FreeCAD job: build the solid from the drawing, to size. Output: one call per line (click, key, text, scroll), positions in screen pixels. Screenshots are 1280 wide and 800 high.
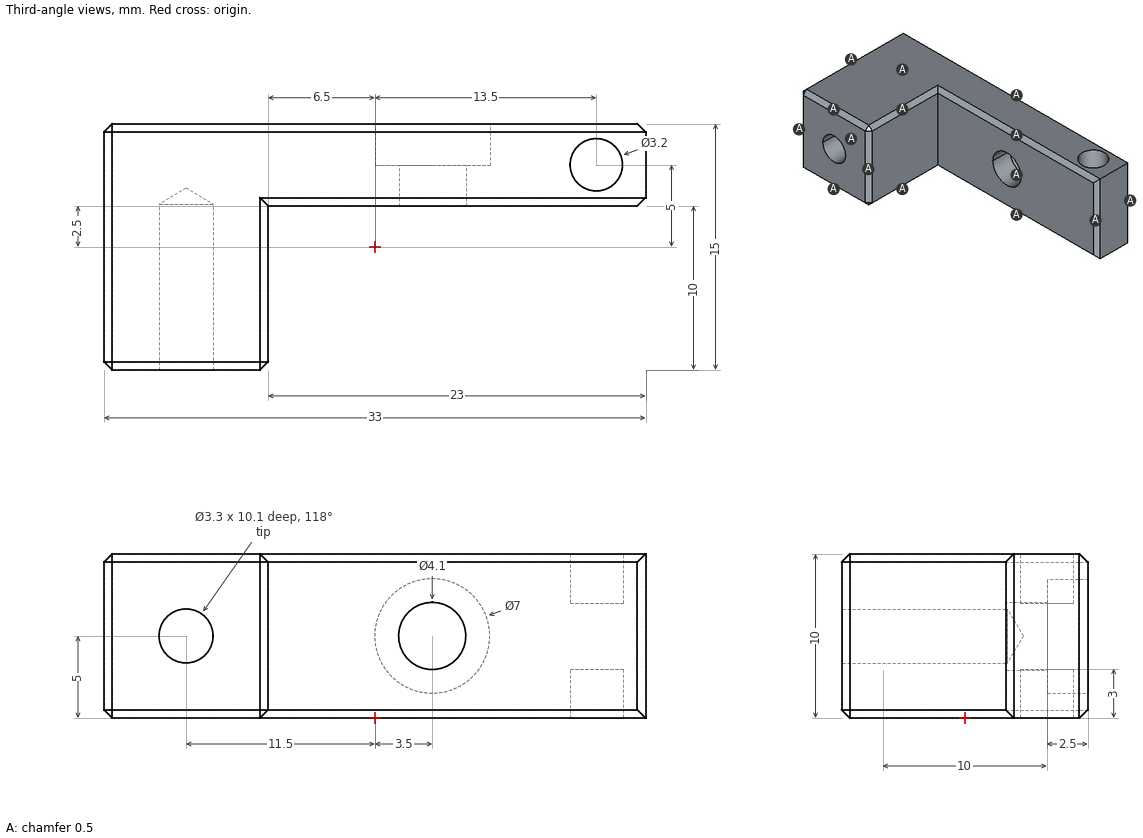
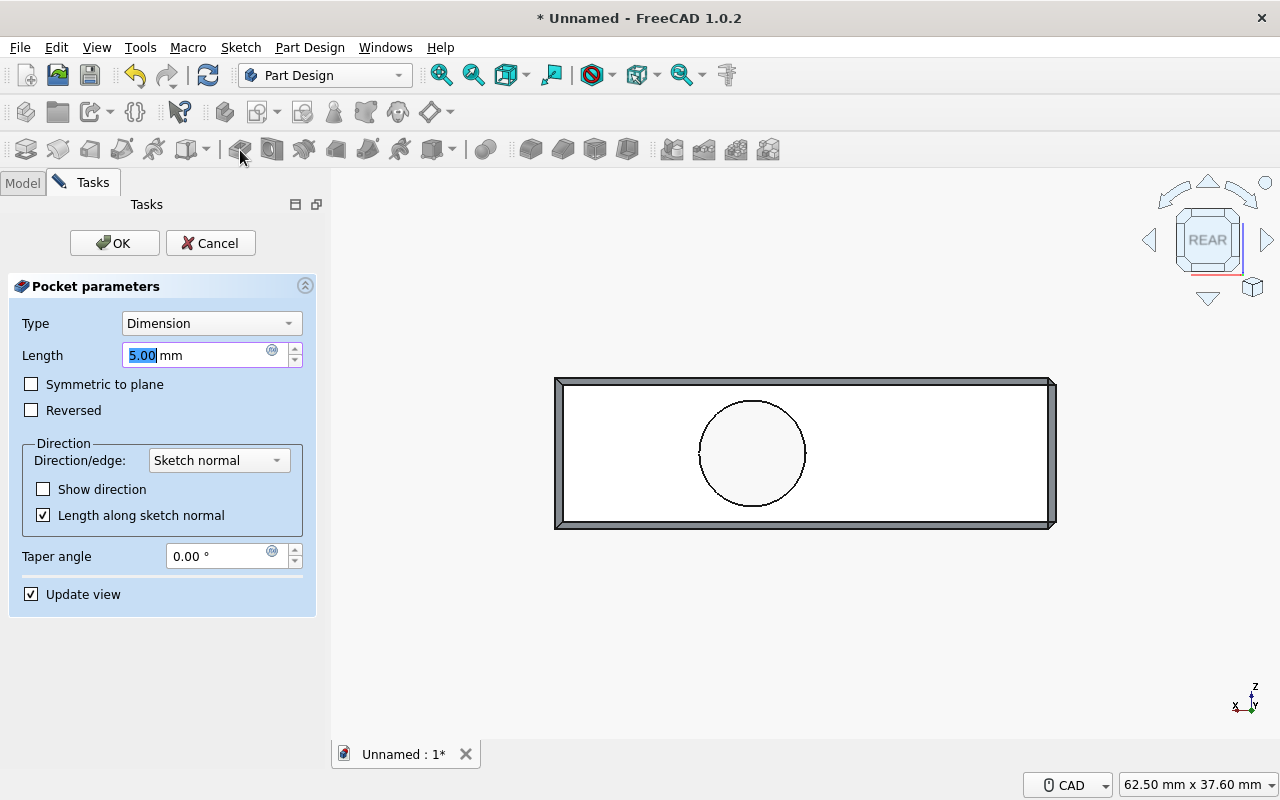
text(2.5)
key(Tab)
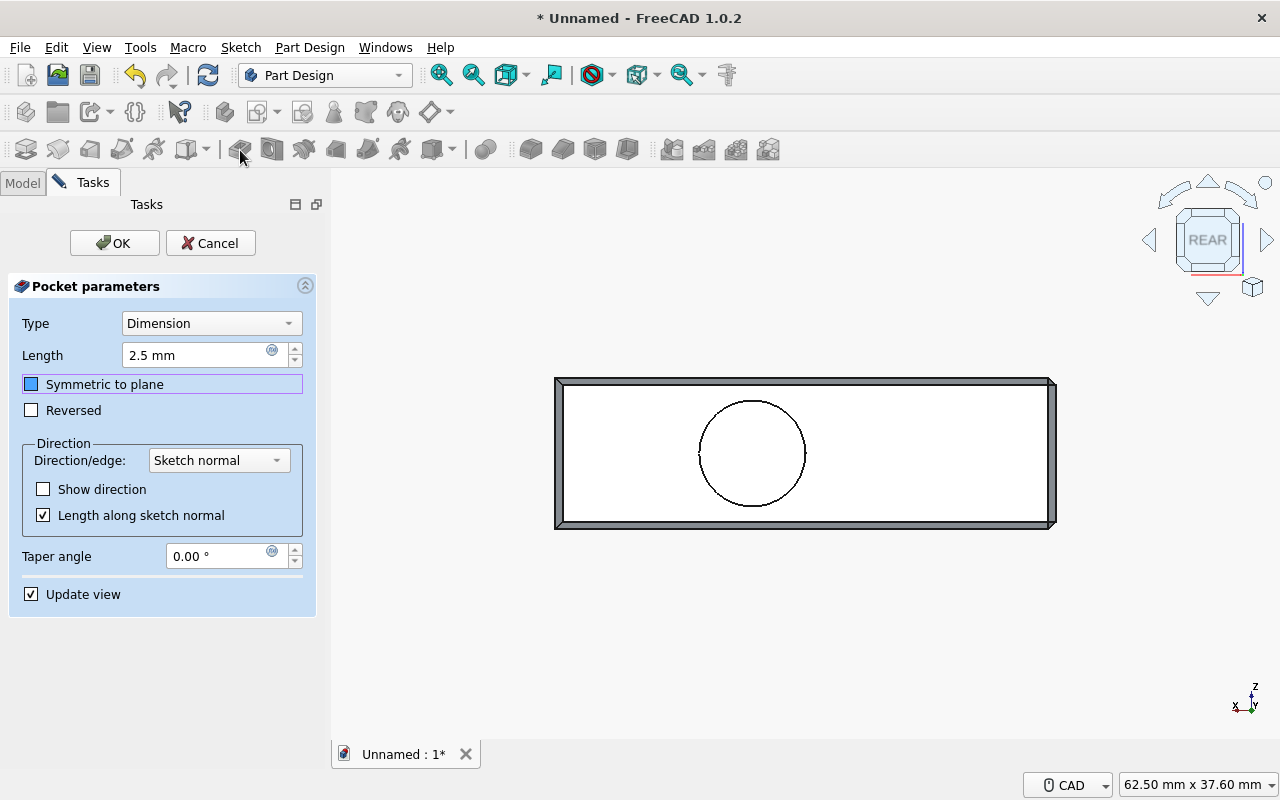
click(115, 243)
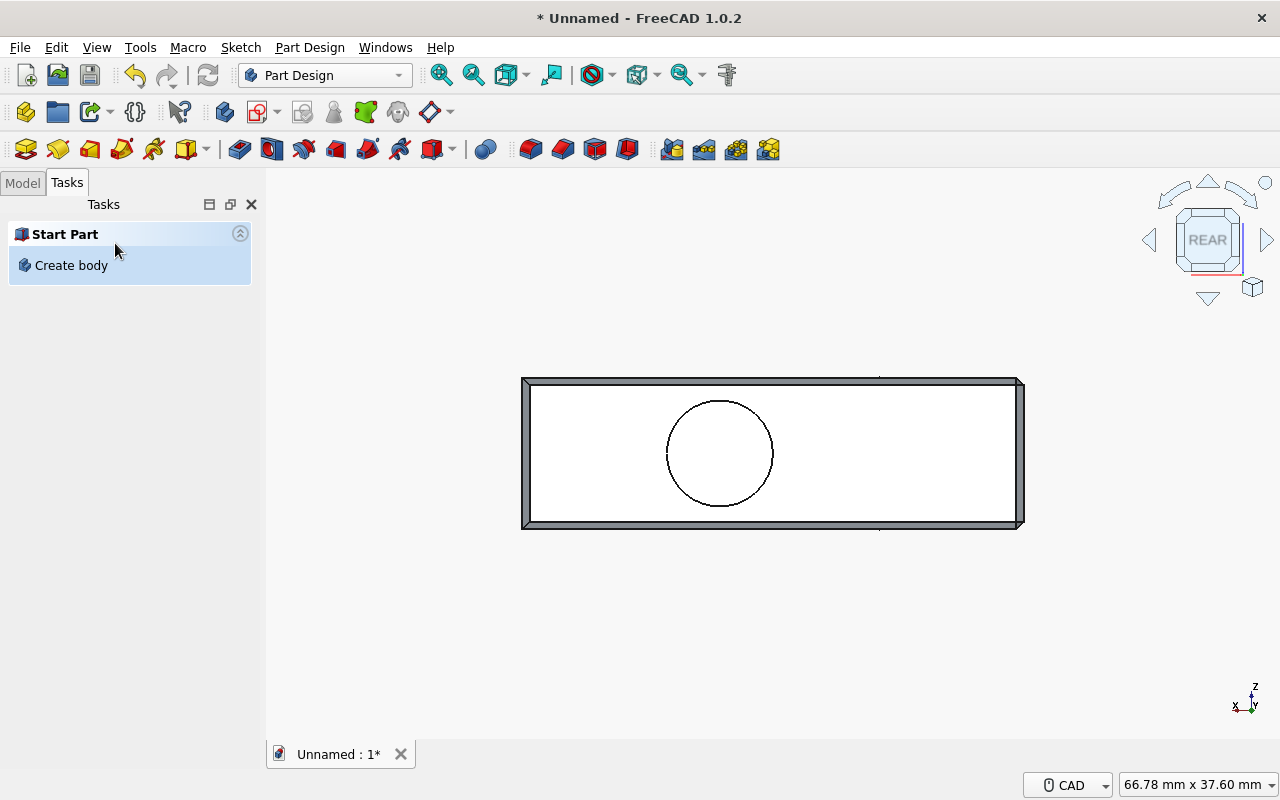
click(258, 112)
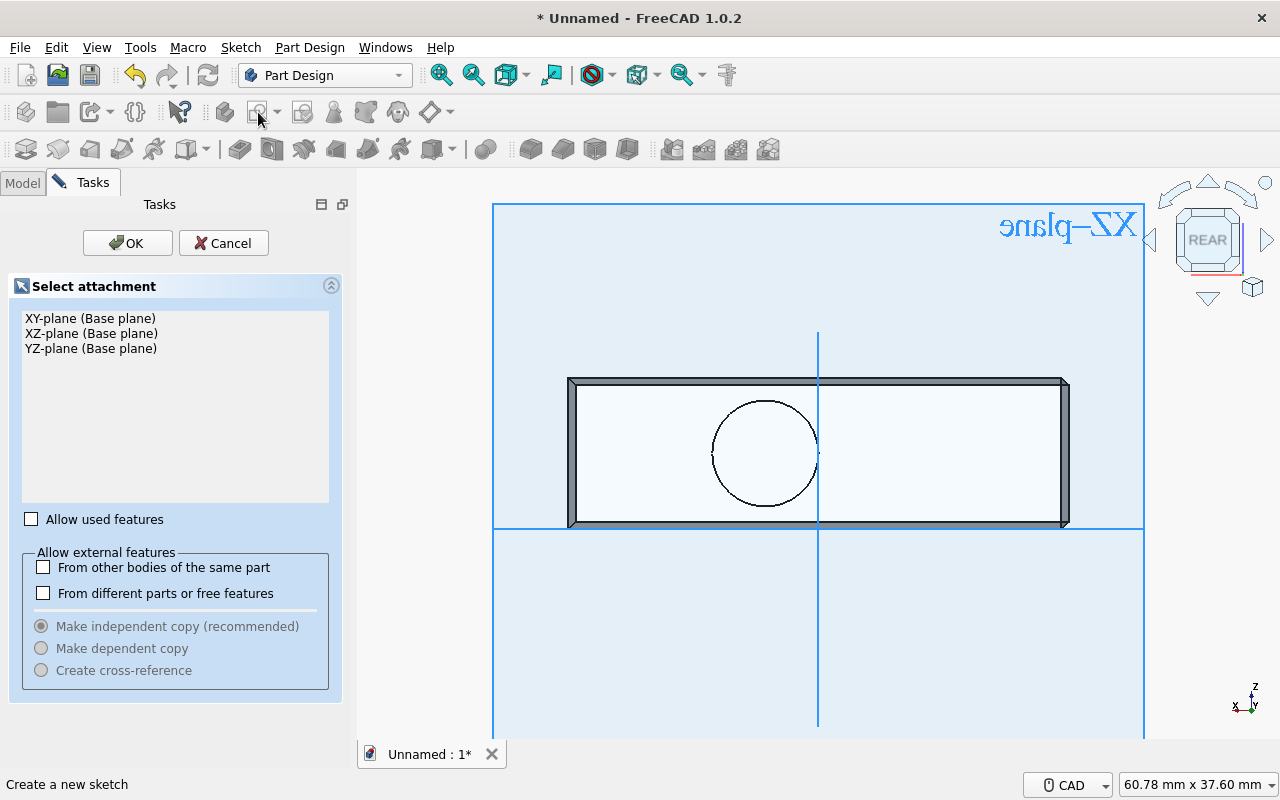
click(82, 318)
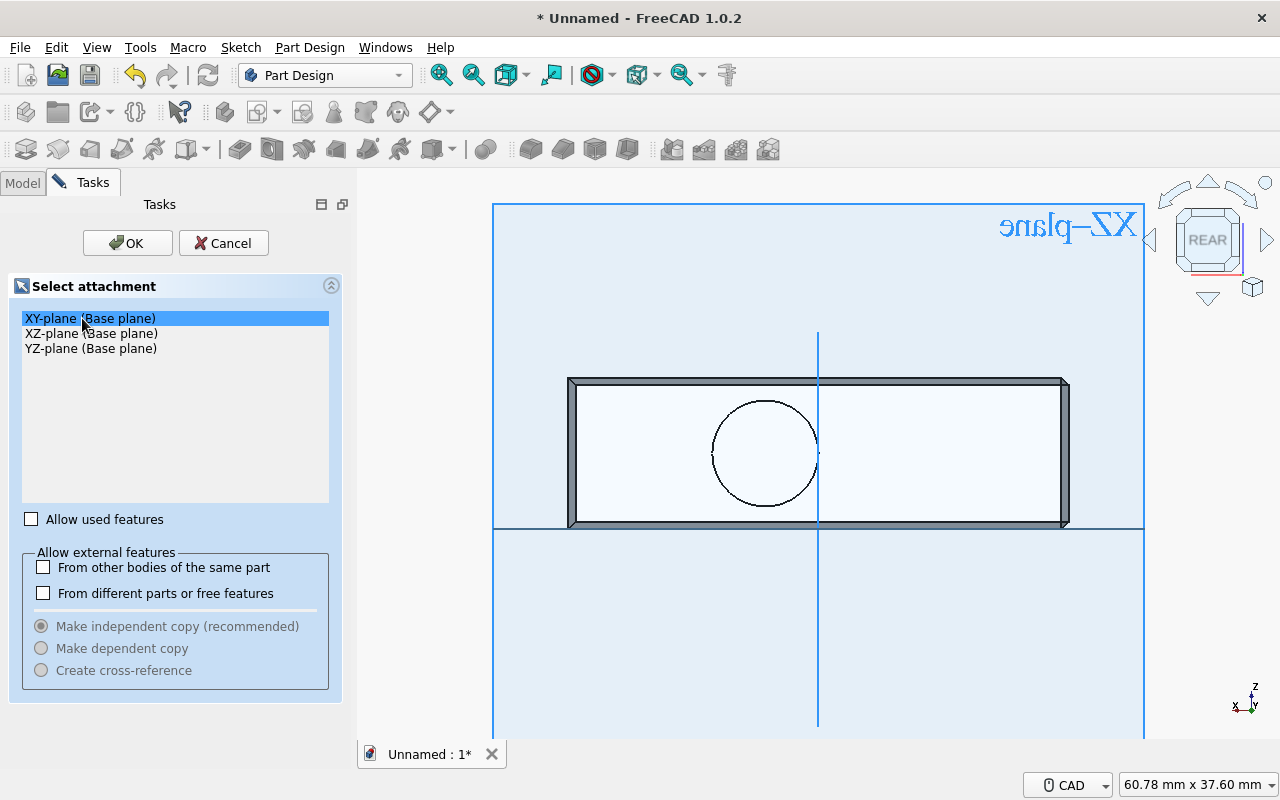
click(128, 243)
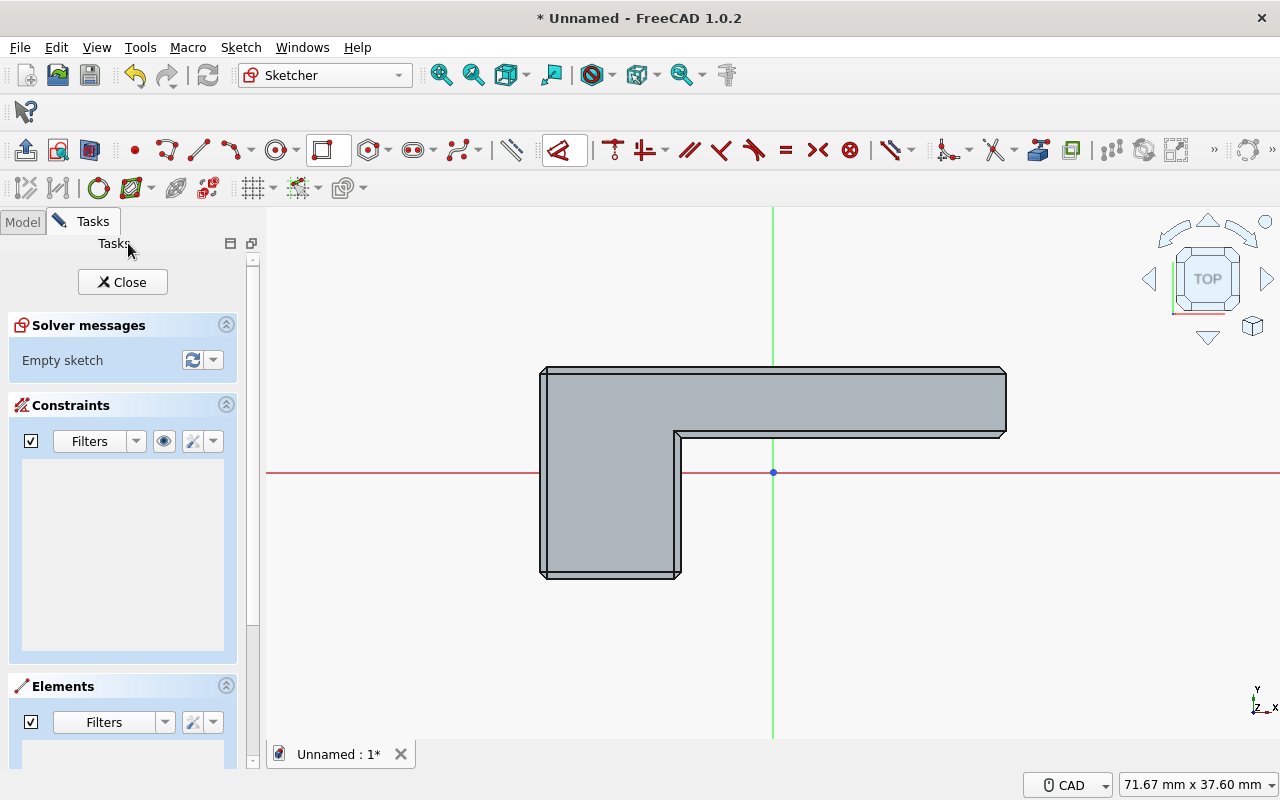
click(90, 150)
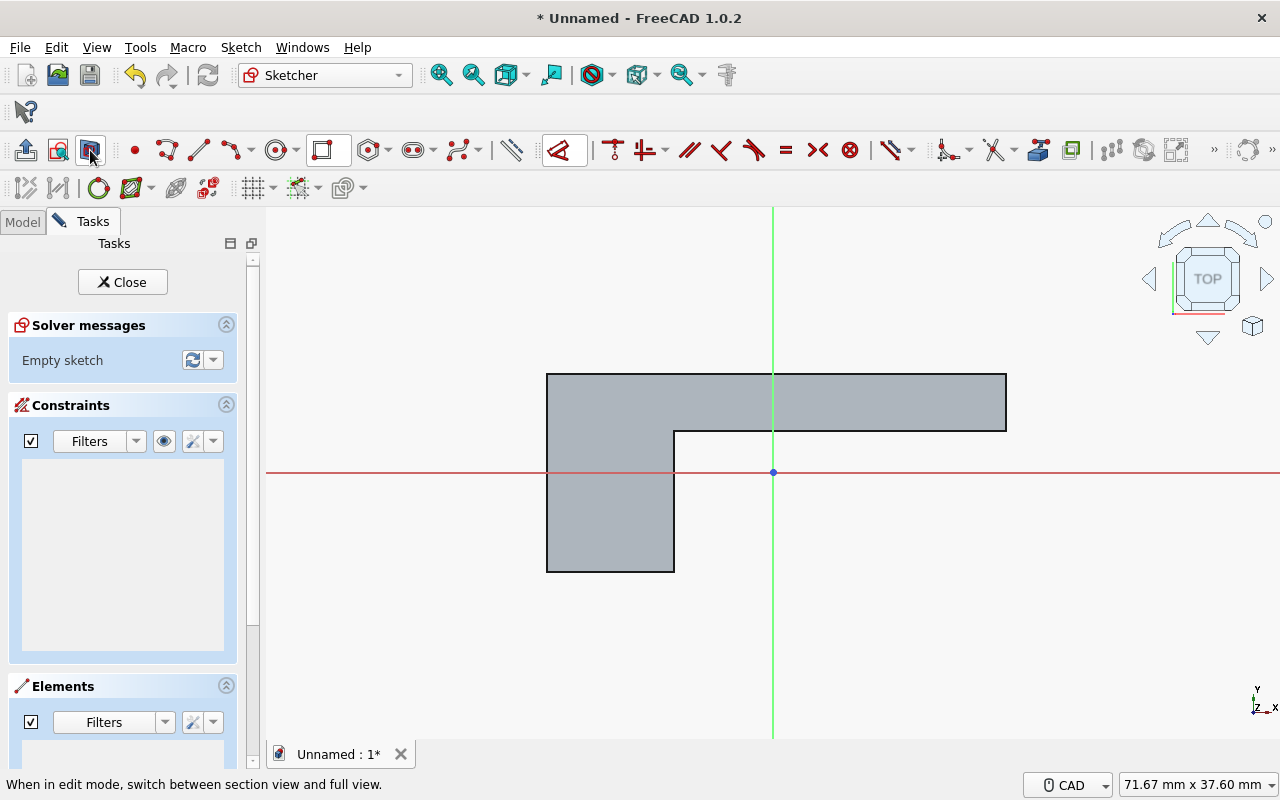
scroll(1005, 391, up, 10)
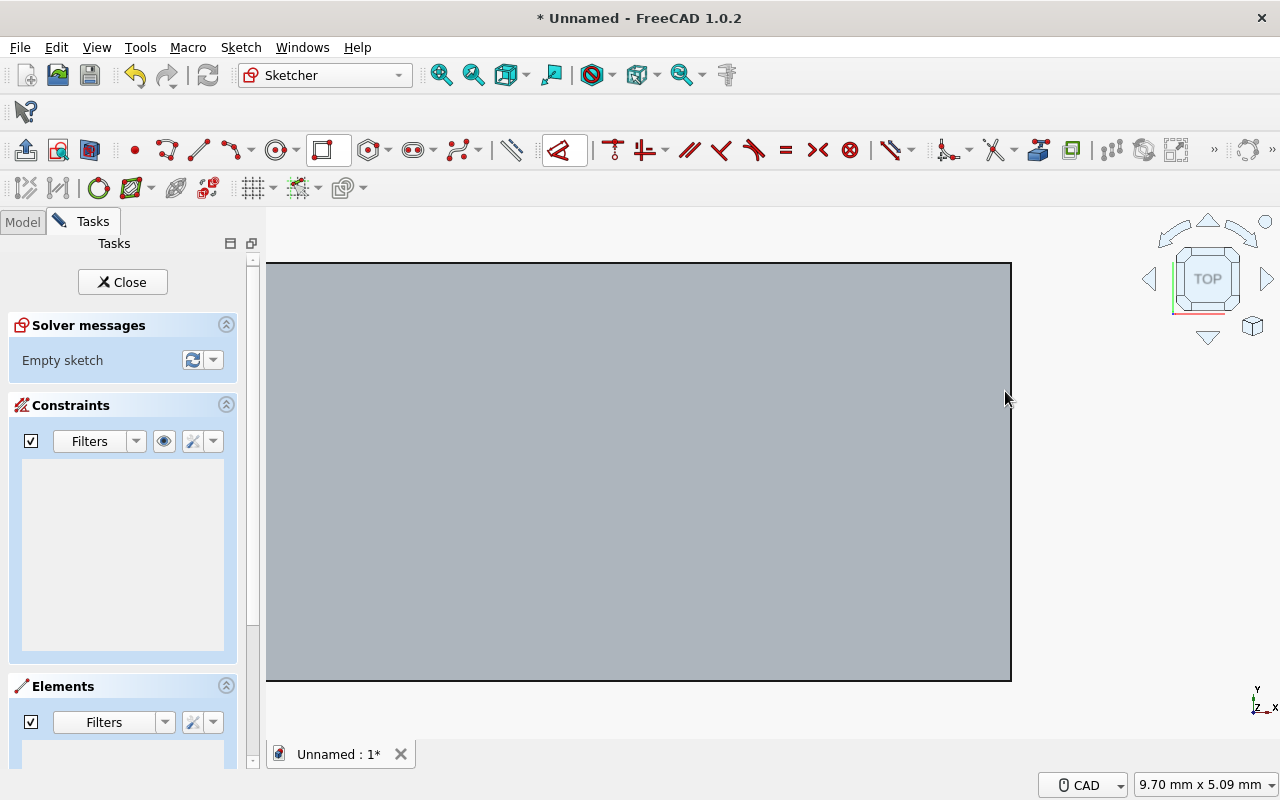
click(276, 150)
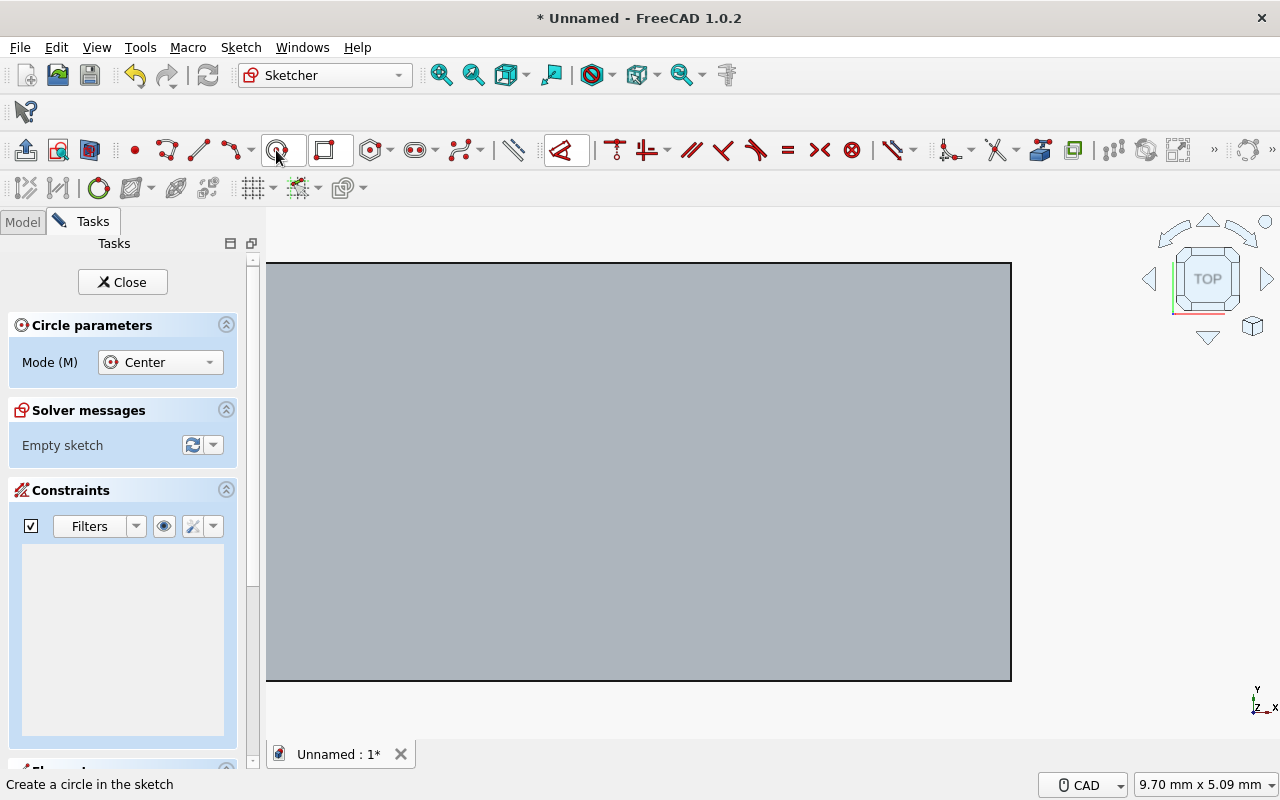
click(697, 472)
move(816, 354)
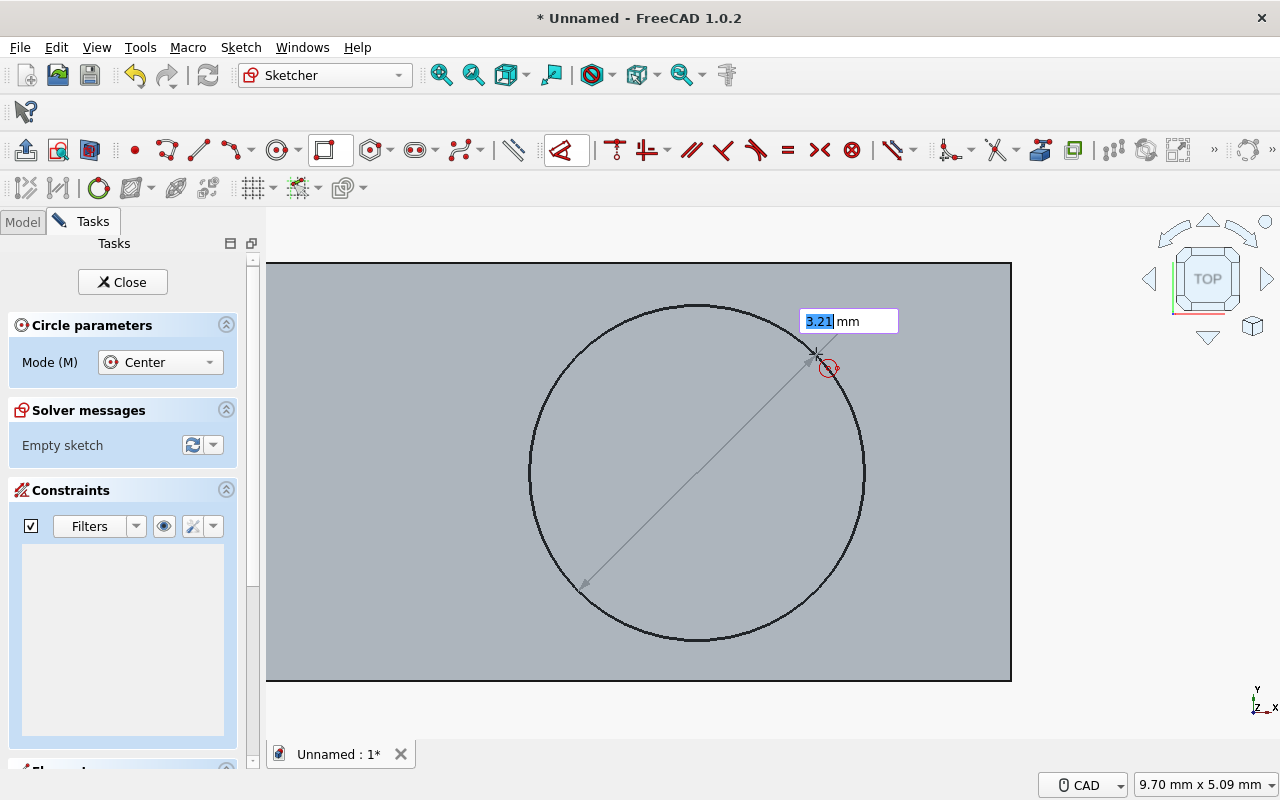
text(3.2)
key(Return)
key(Escape)